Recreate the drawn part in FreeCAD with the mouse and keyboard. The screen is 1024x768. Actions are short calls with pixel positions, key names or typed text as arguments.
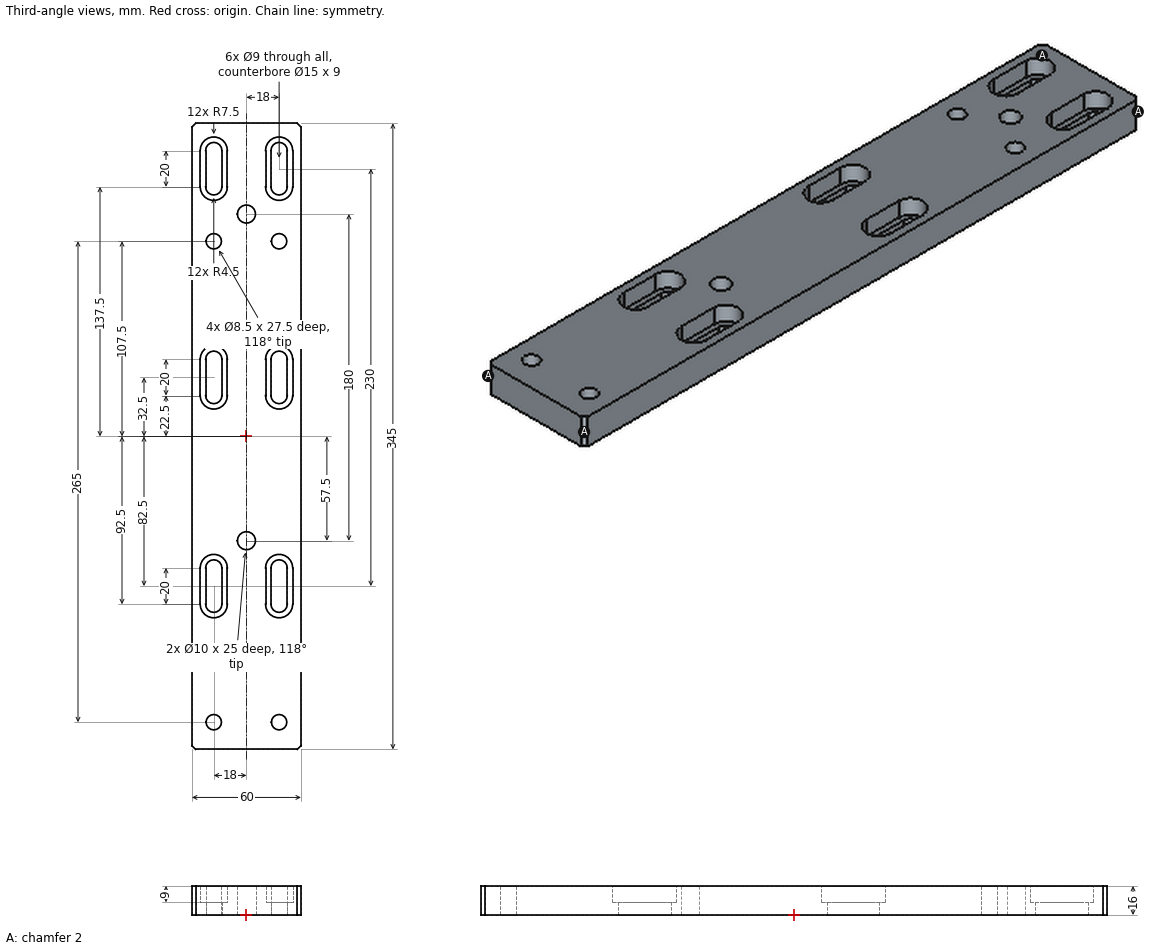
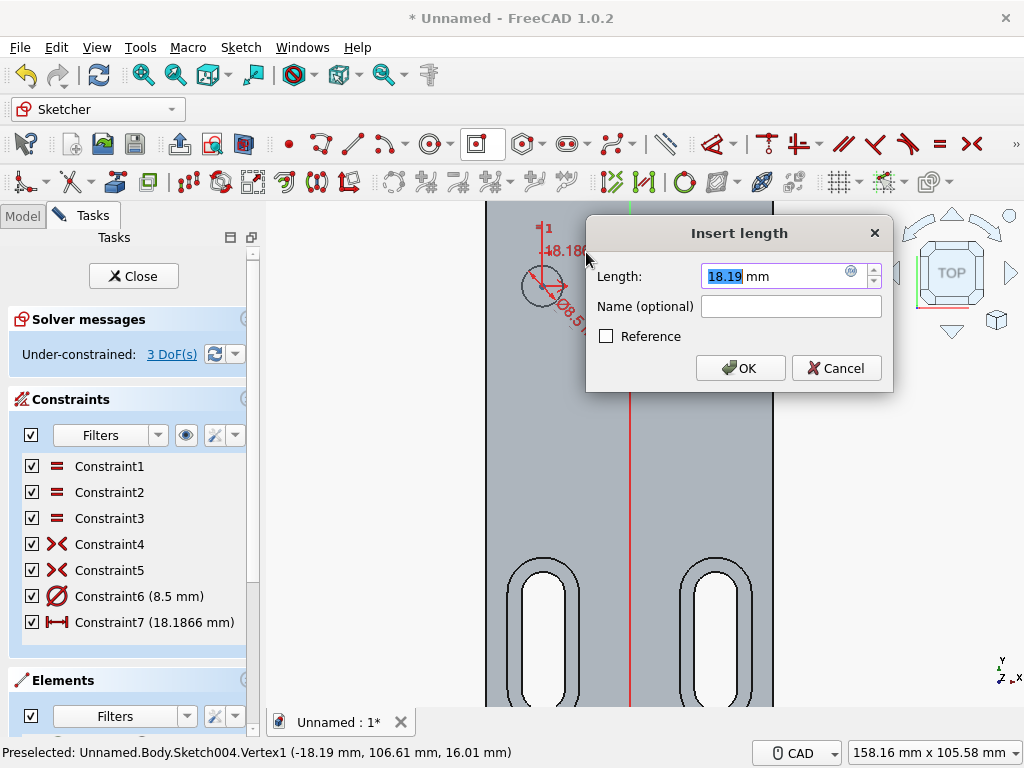
text(18)
key(Return)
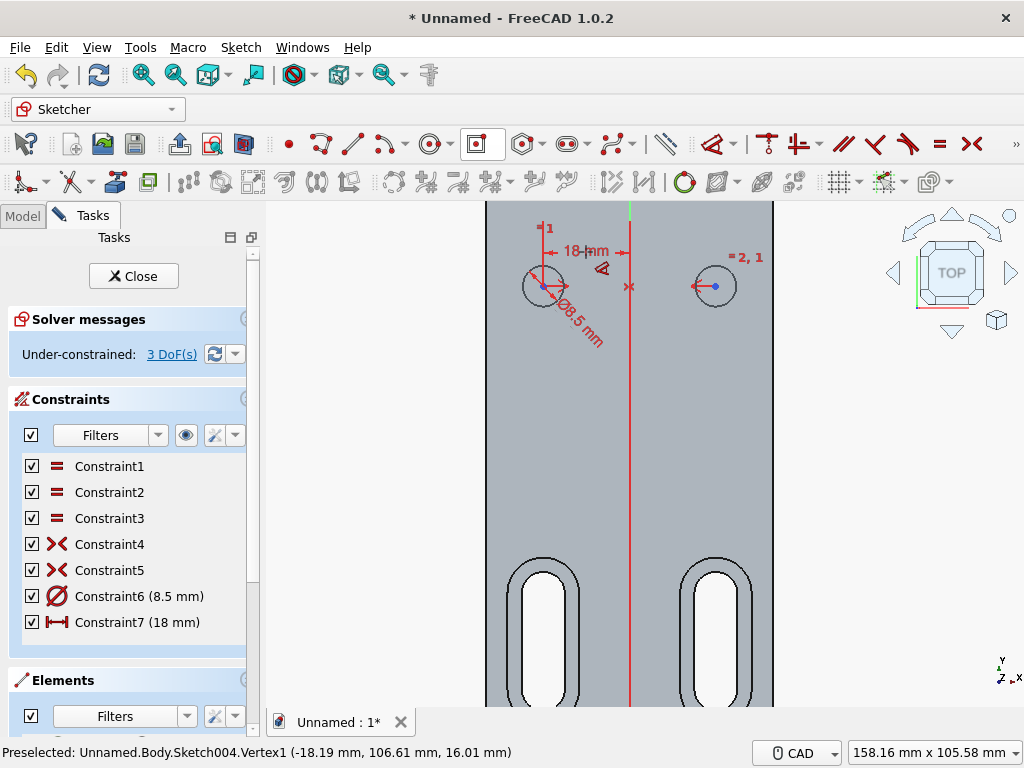
scroll(559, 302, down, 7)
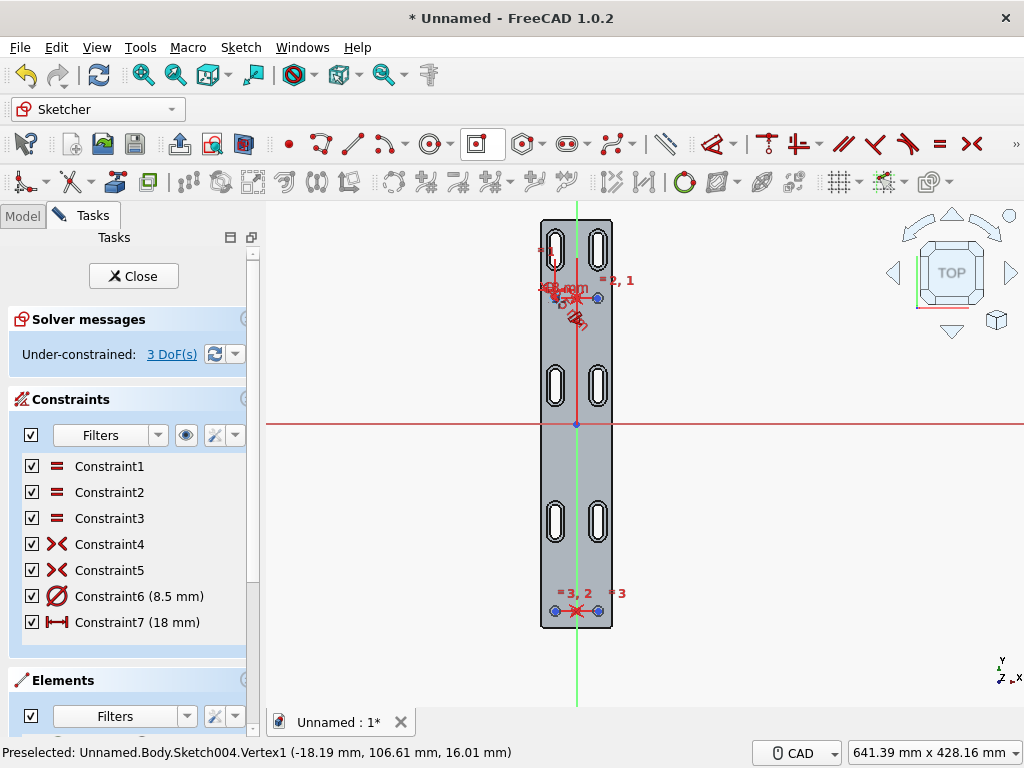
scroll(555, 611, up, 4)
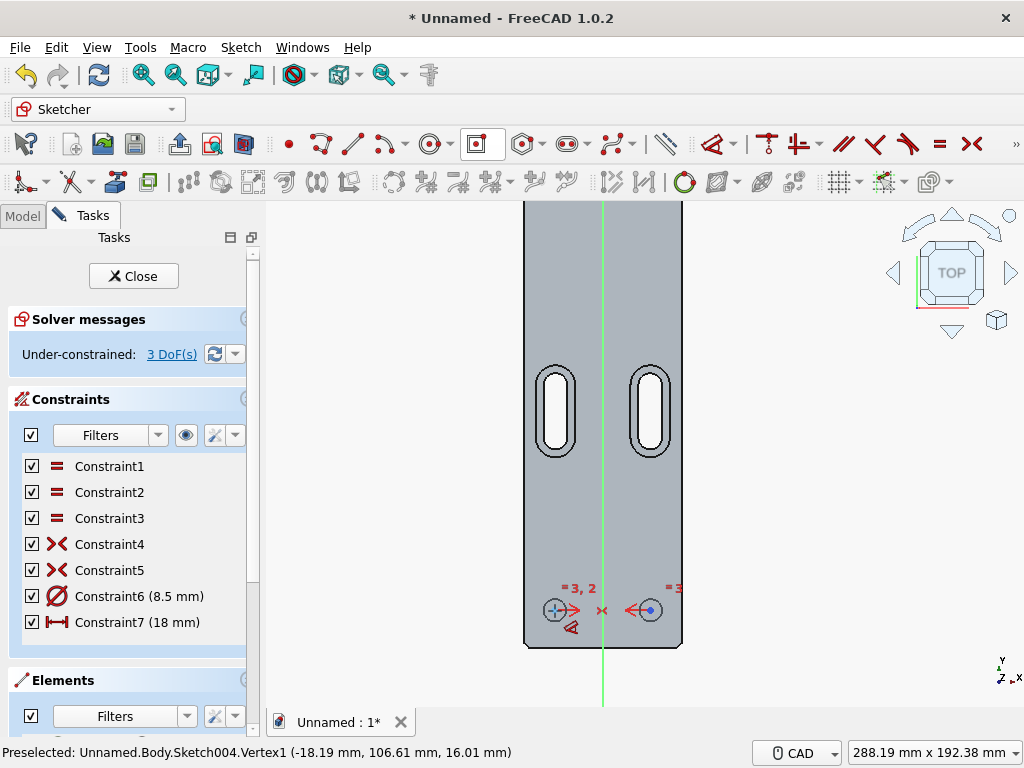
click(555, 610)
click(579, 644)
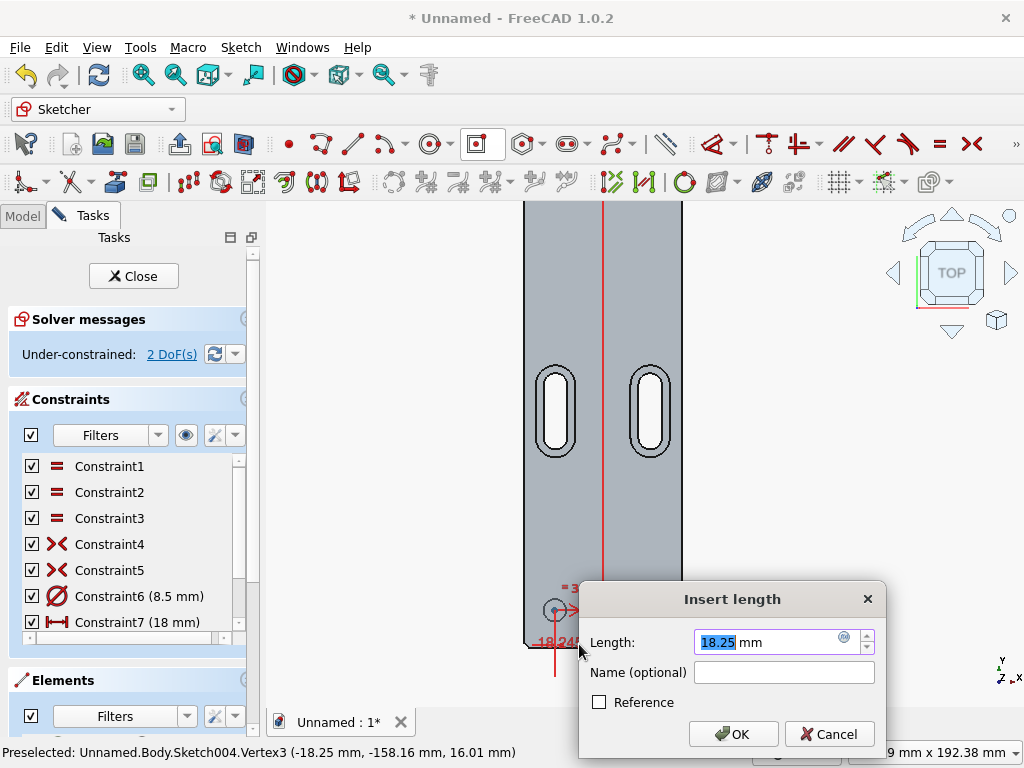
text(18)
key(Return)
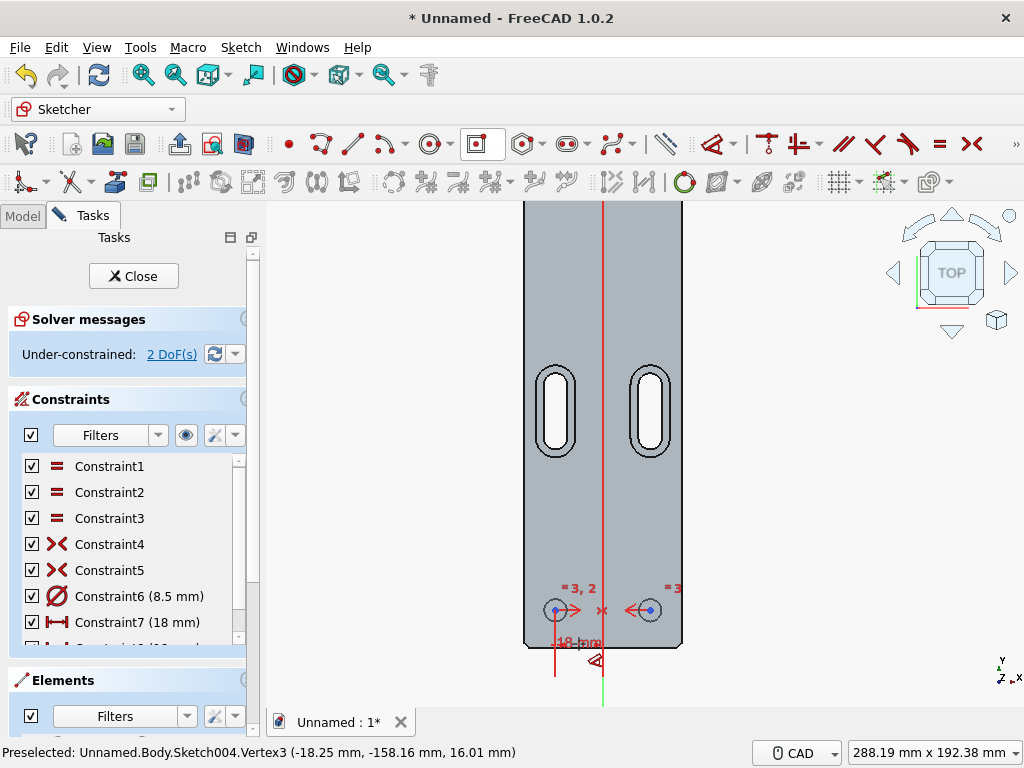
scroll(555, 612, down, 4)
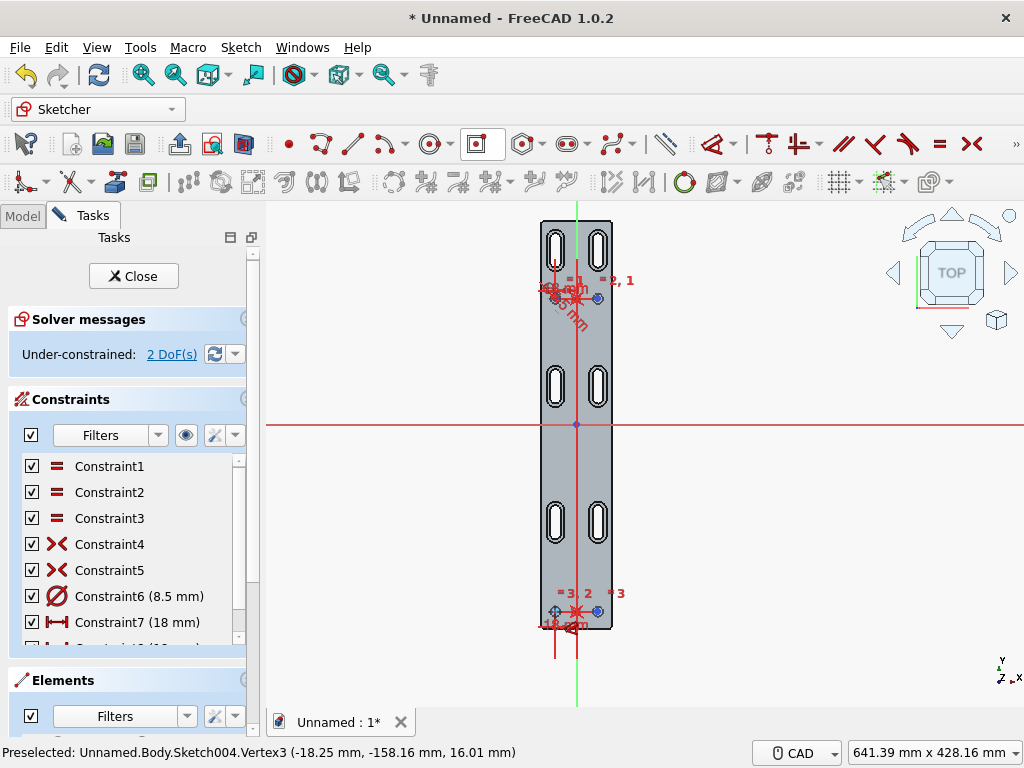
click(555, 299)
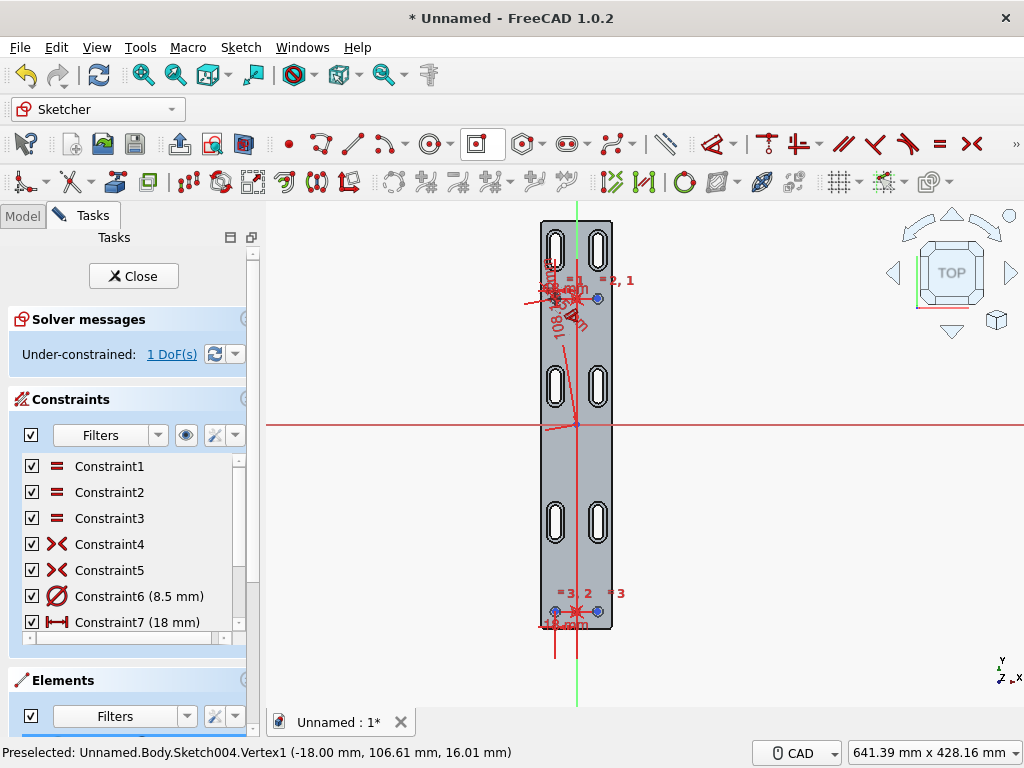
click(555, 612)
click(521, 455)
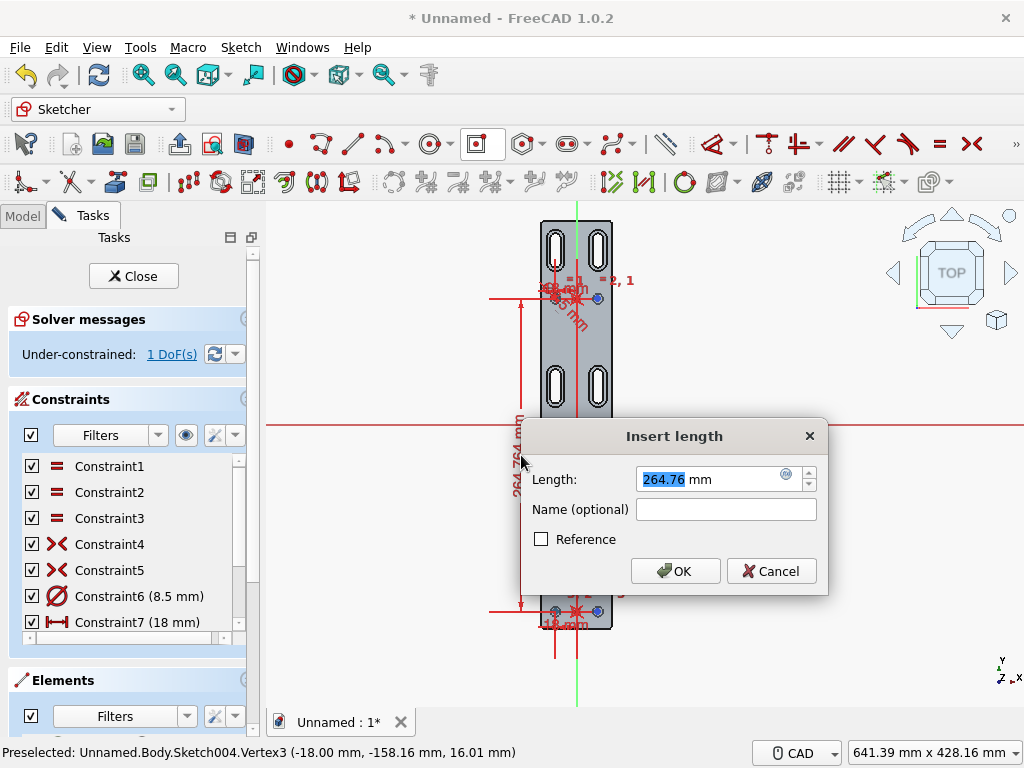
text(265)
key(Return)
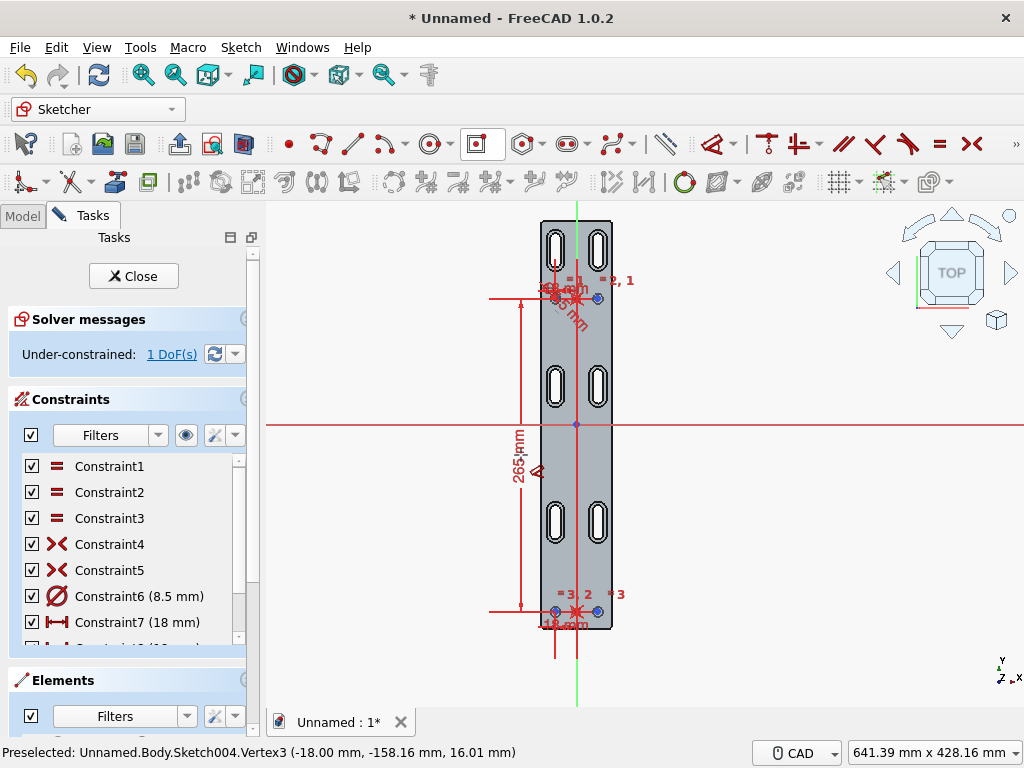
click(555, 299)
click(521, 362)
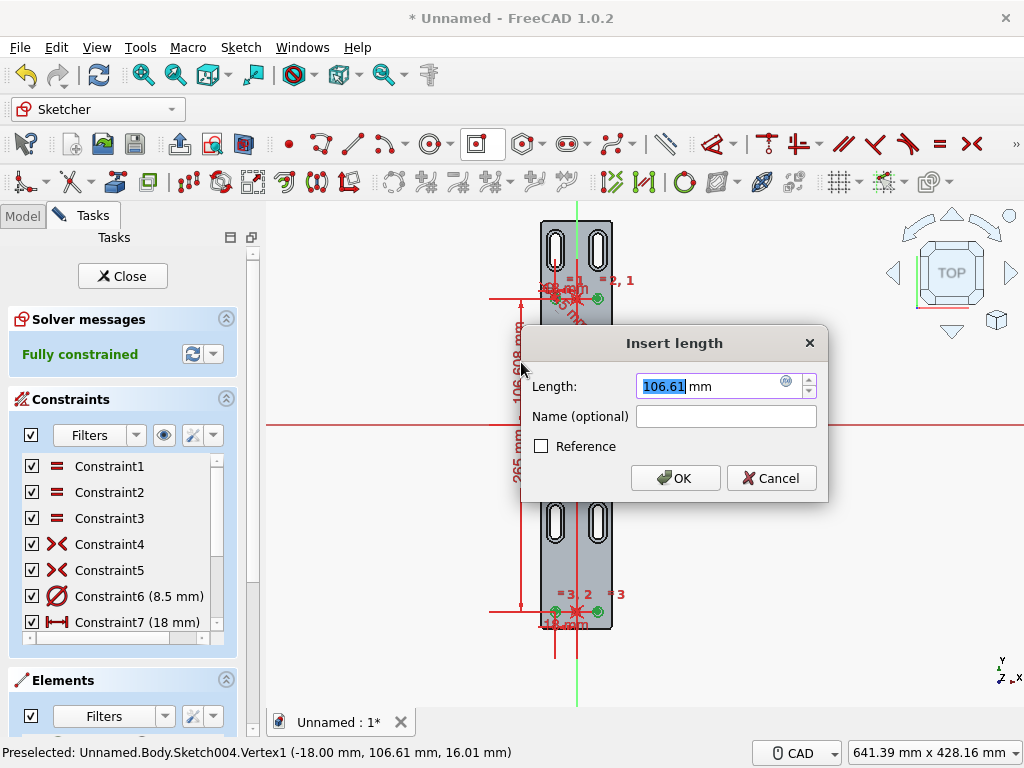
text(107.5)
key(Return)
key(Escape)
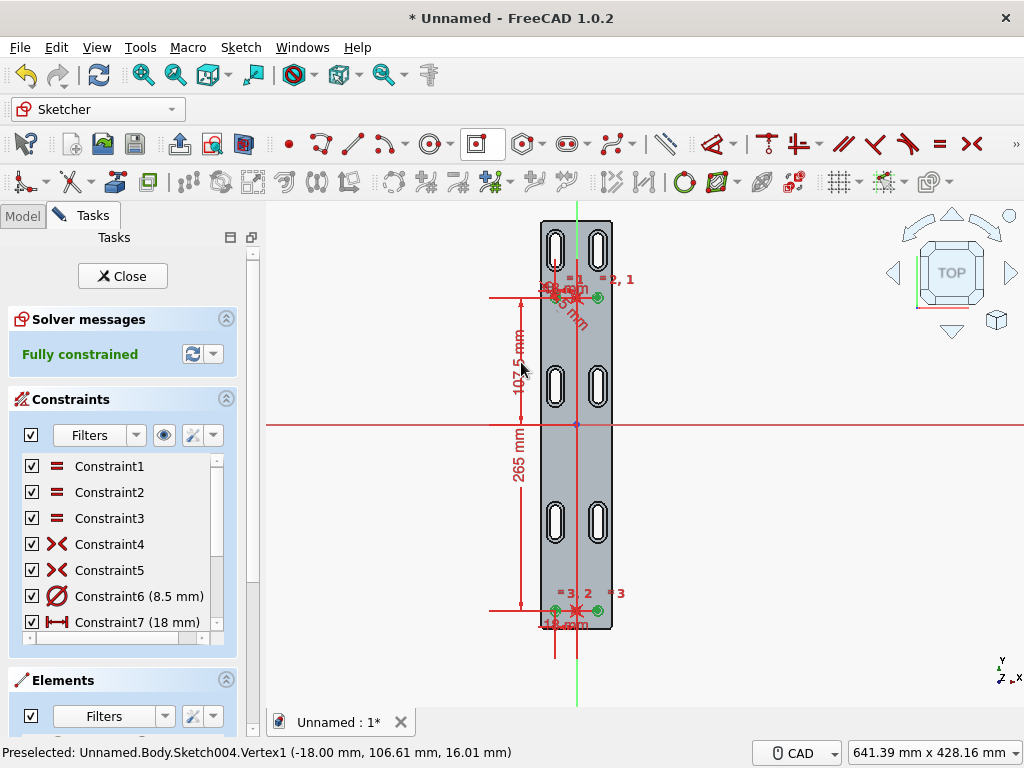
click(123, 276)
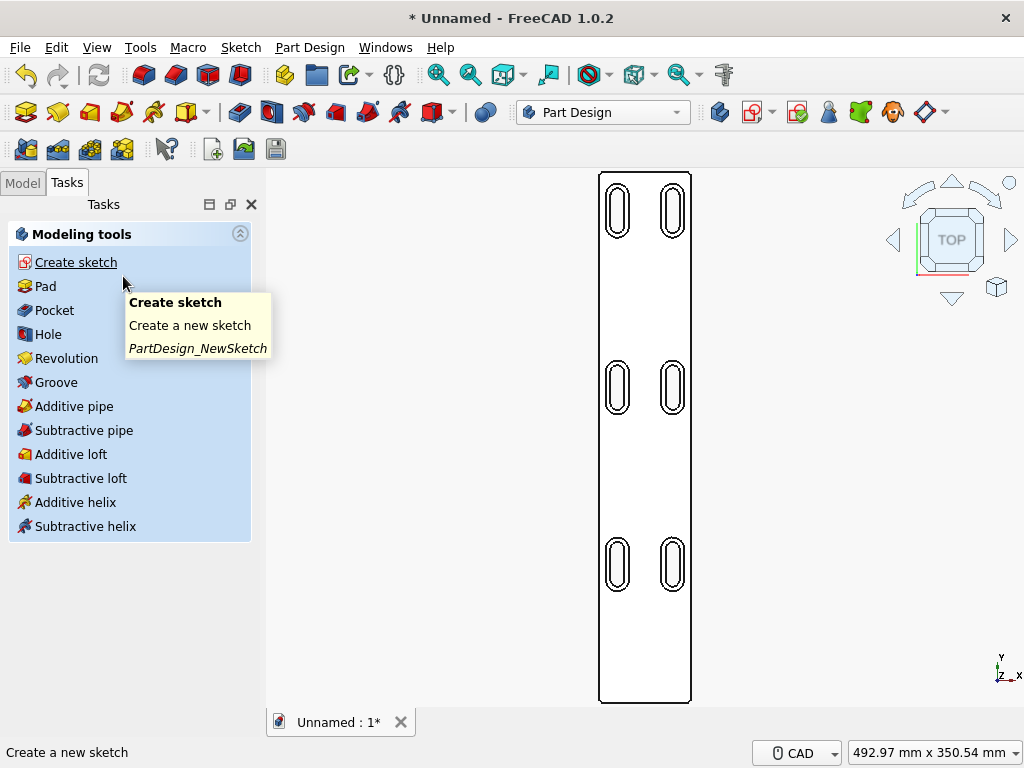
click(272, 112)